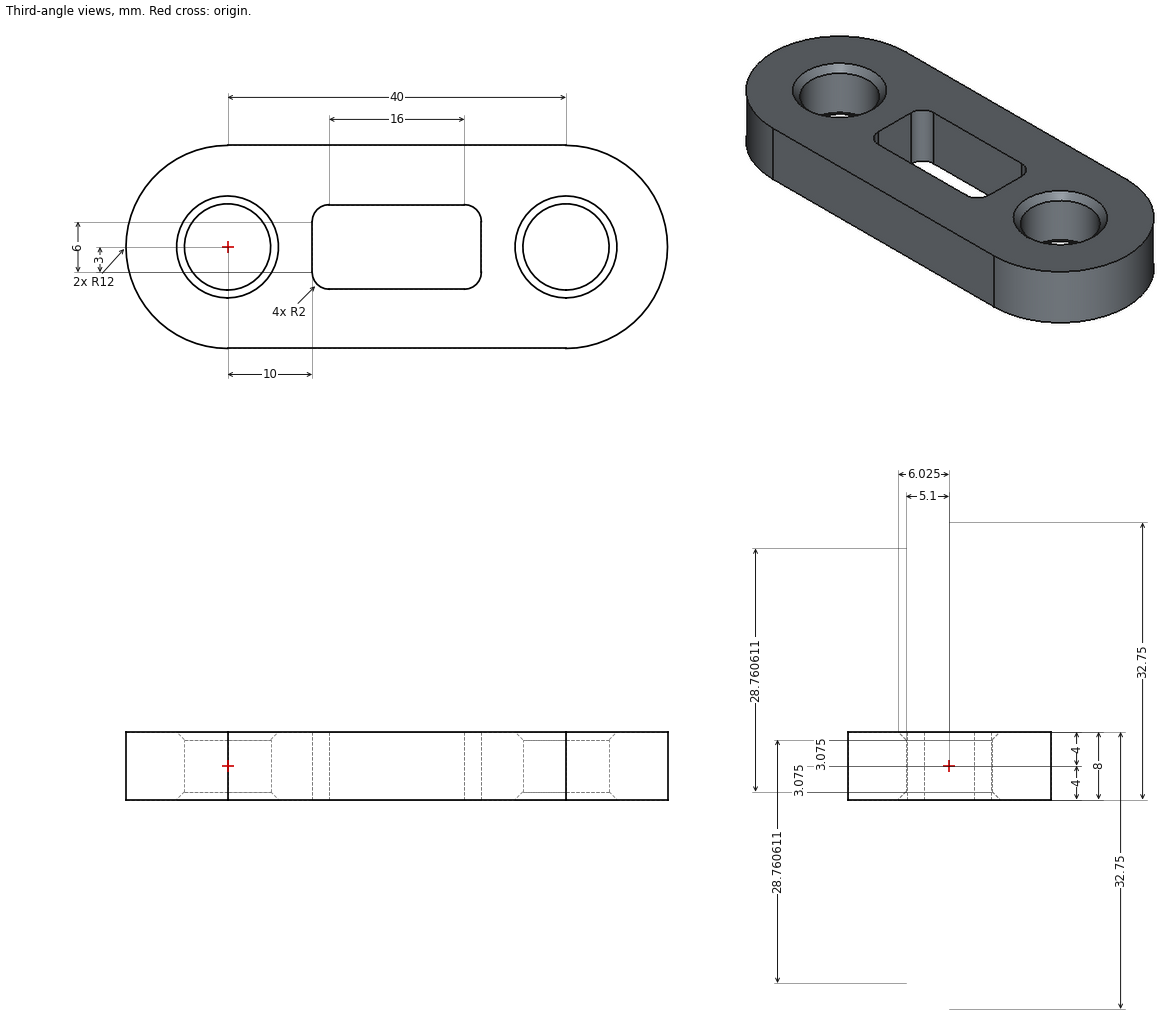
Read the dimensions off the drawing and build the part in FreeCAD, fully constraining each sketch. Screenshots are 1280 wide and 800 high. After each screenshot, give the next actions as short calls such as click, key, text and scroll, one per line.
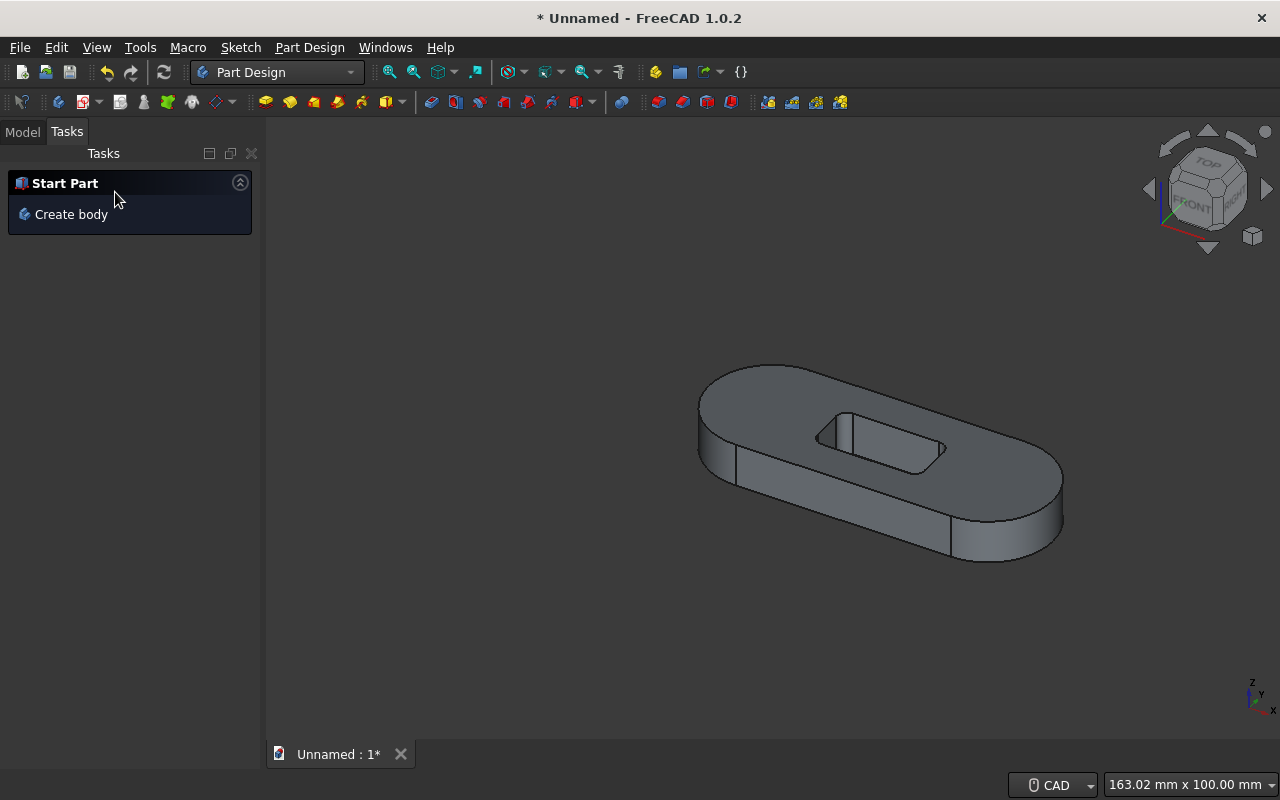
key(v)
key(f)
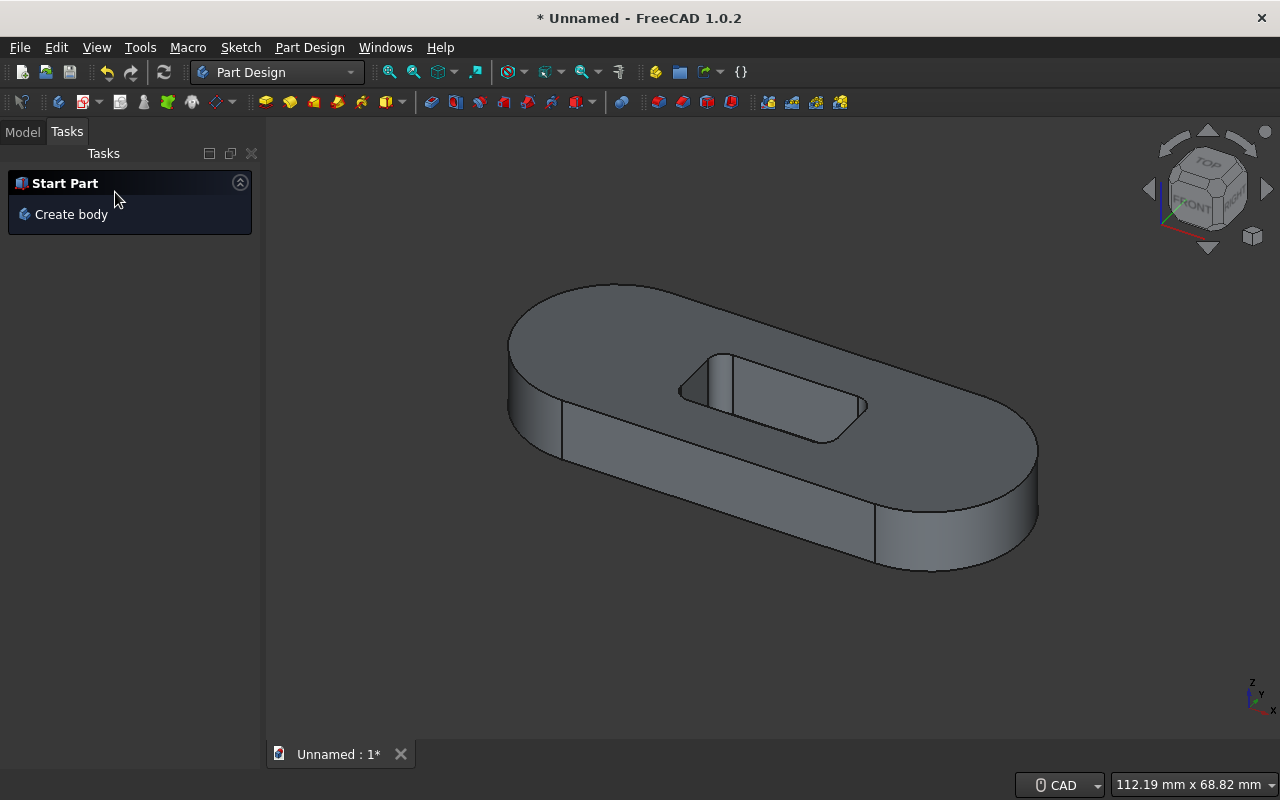
click(84, 102)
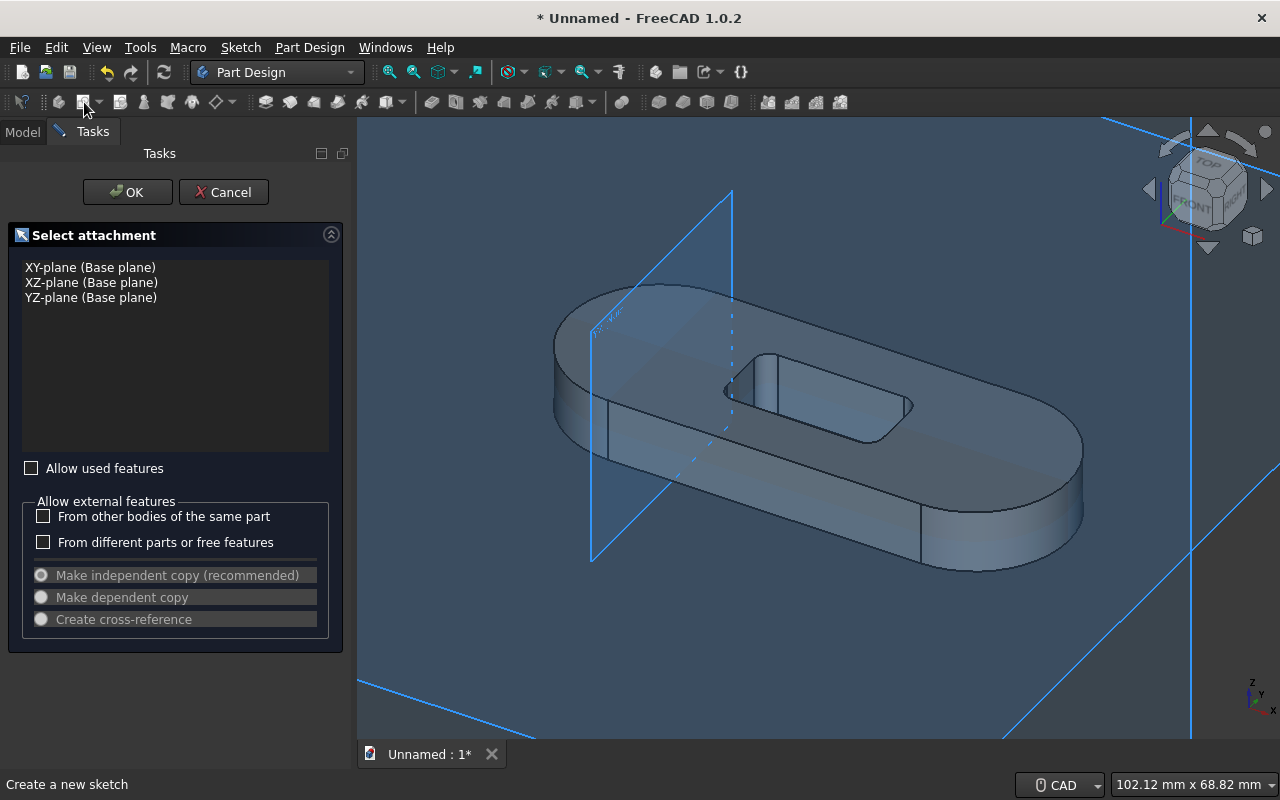
click(82, 298)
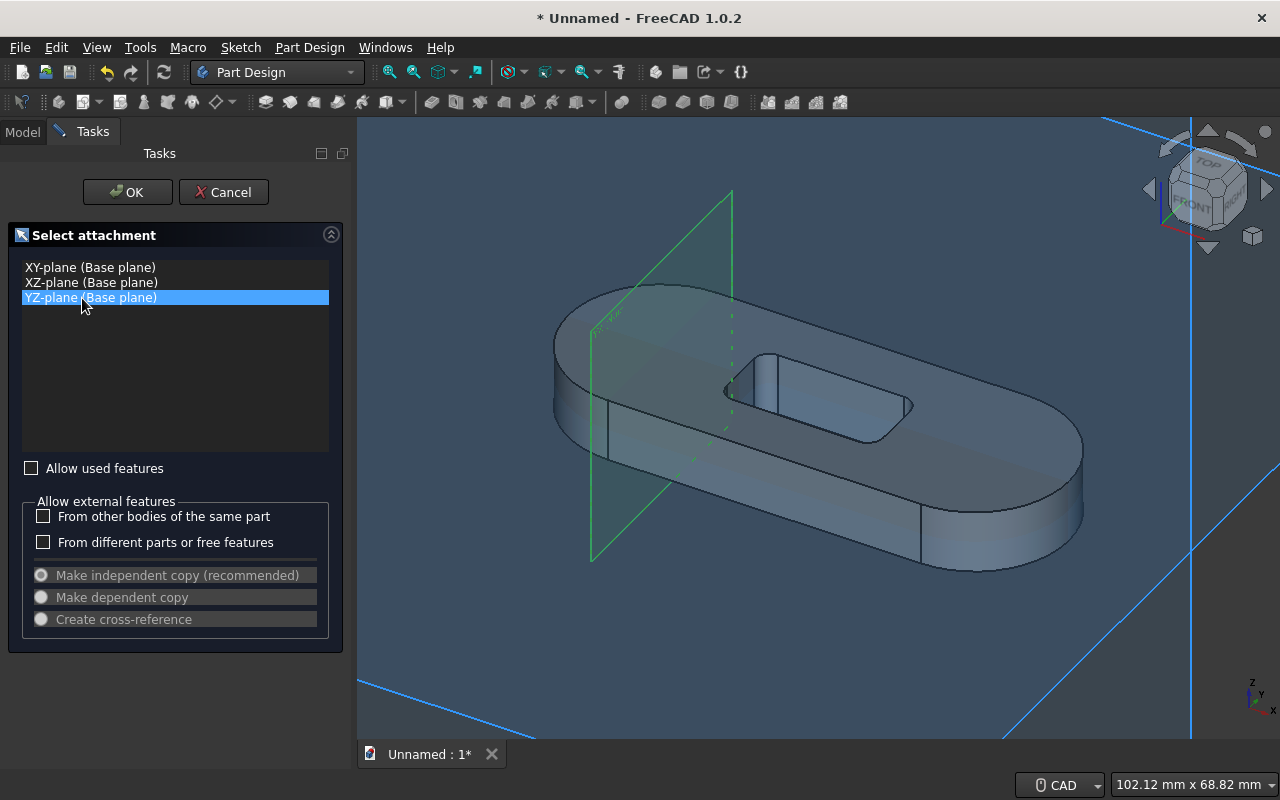
click(128, 192)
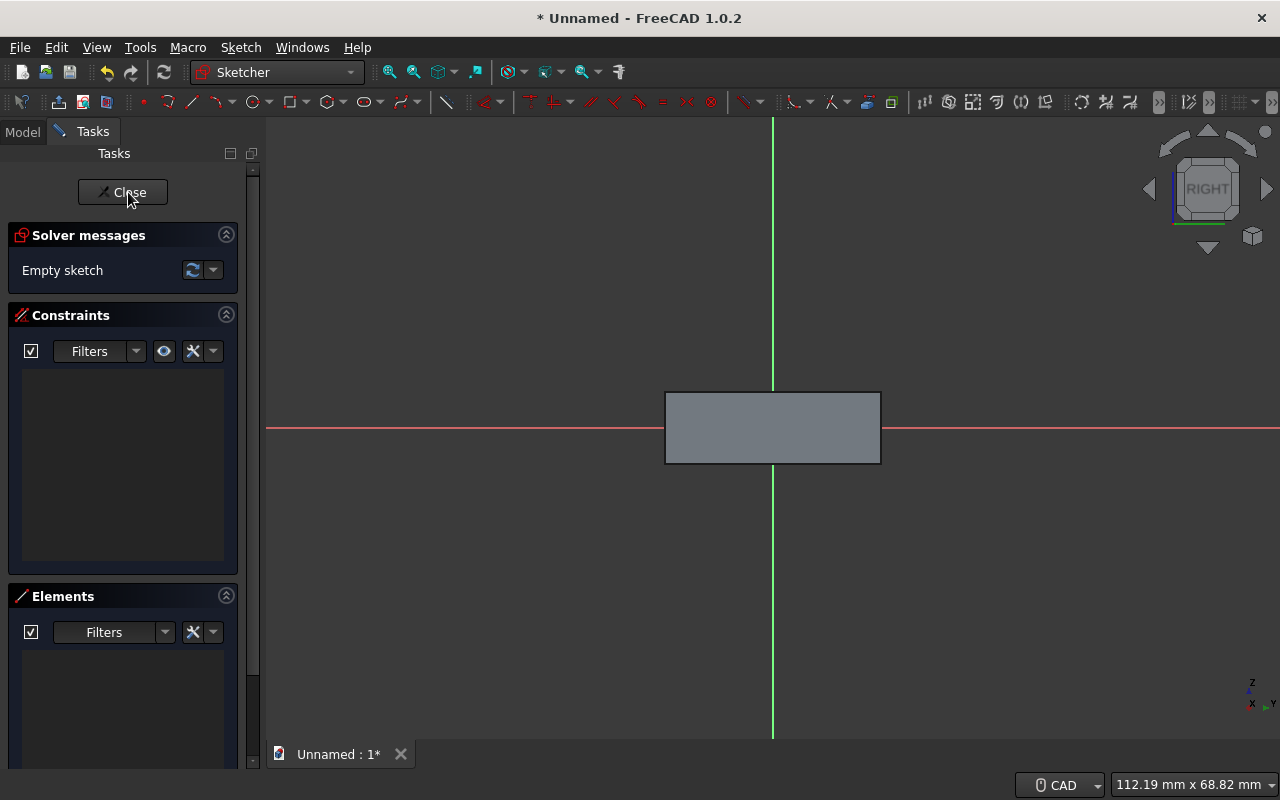
key(q)
key(s)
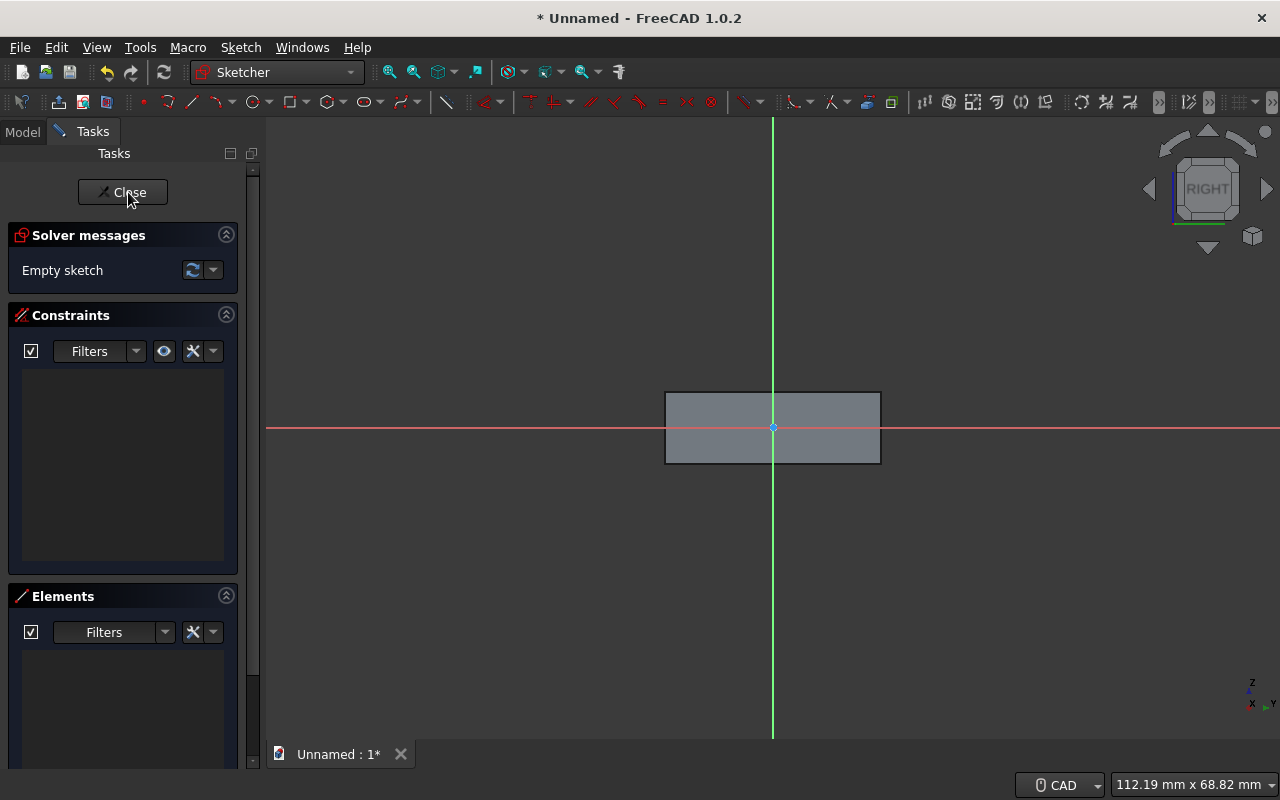
scroll(932, 711, up, 1)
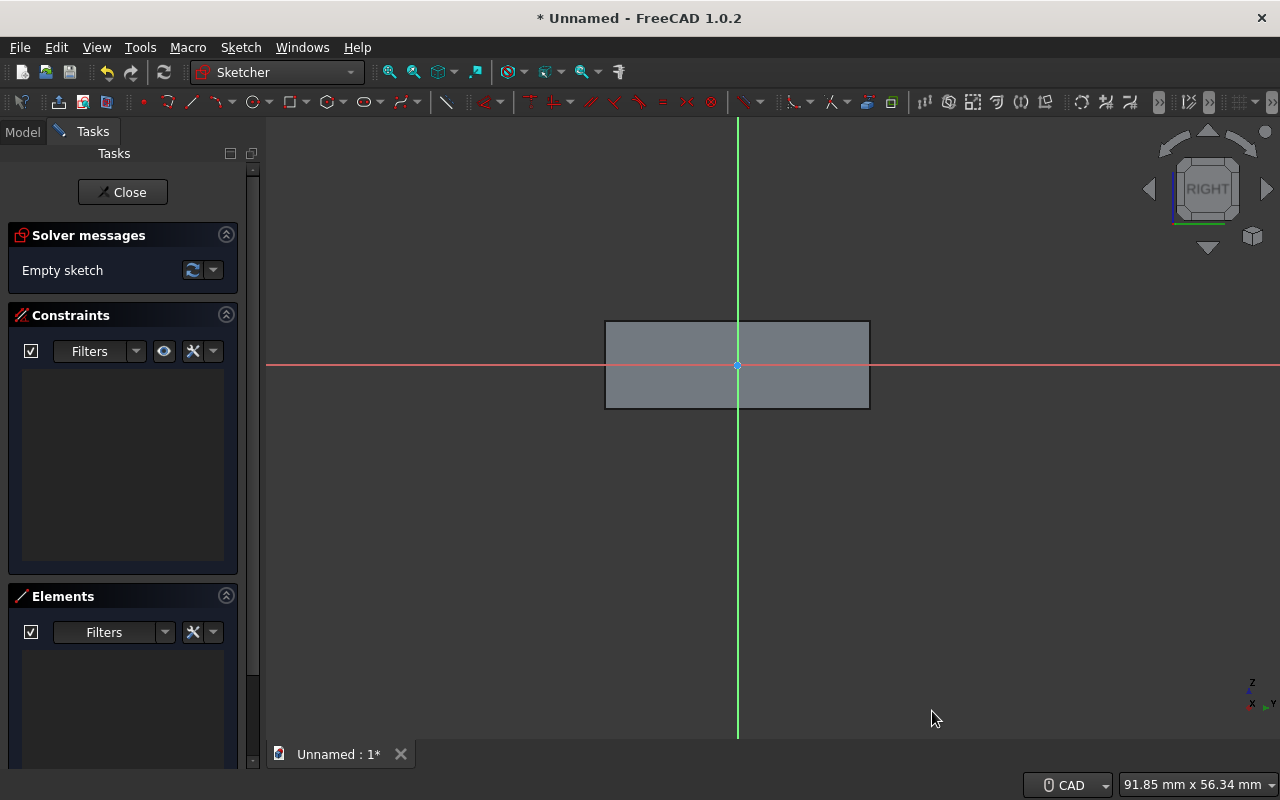
click(168, 102)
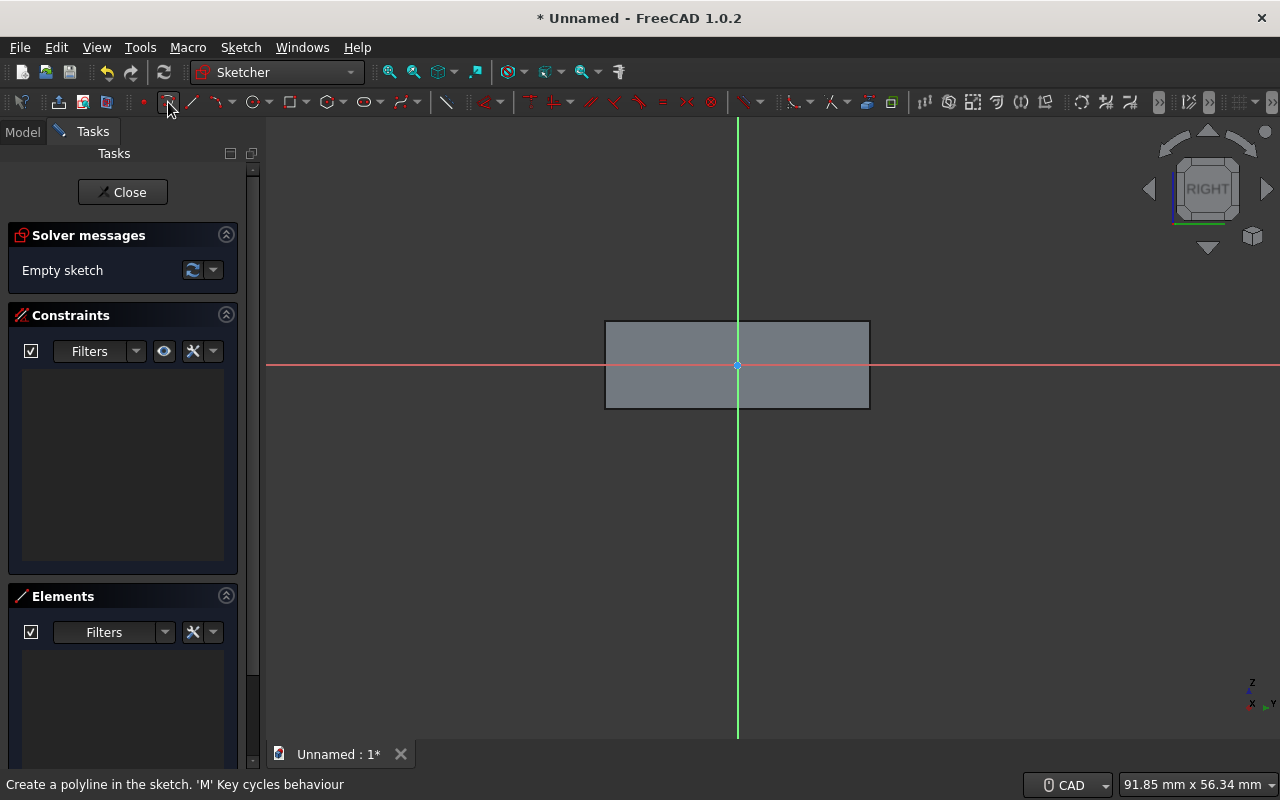
click(738, 321)
click(671, 321)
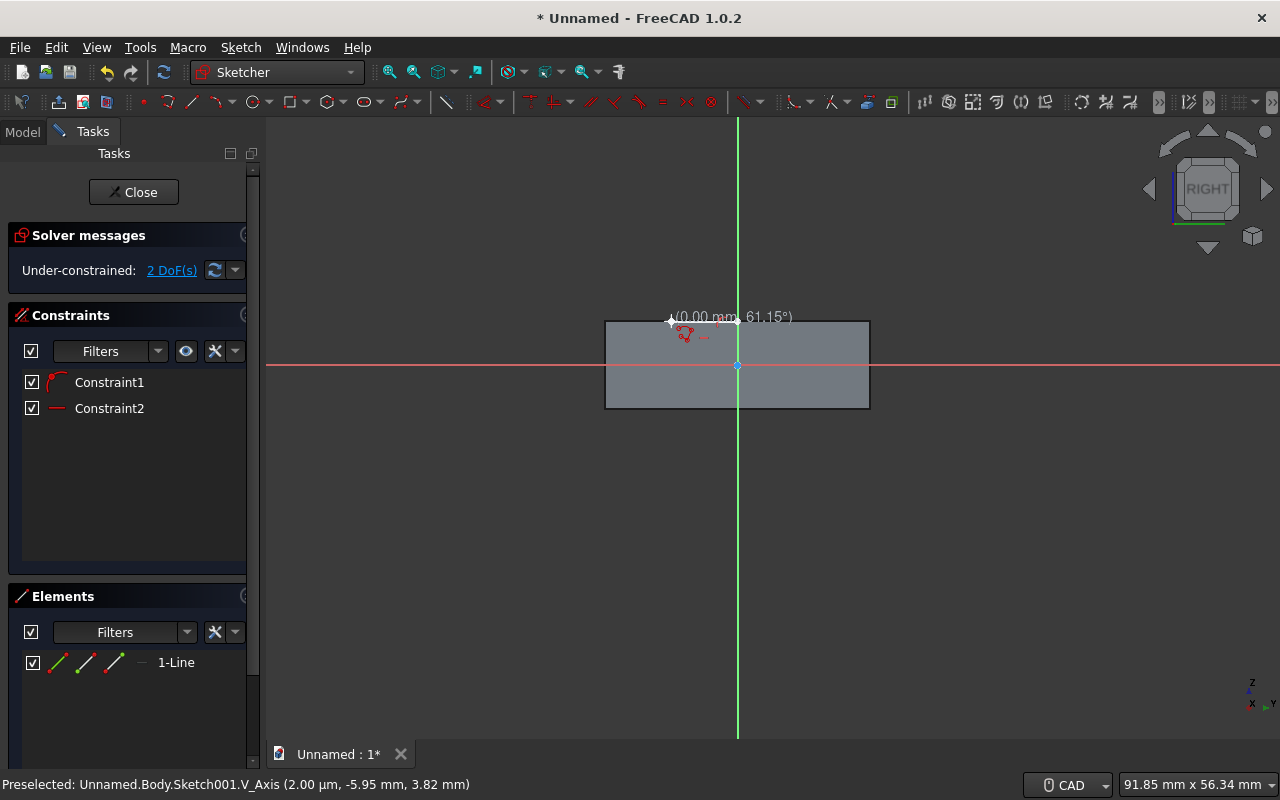
scroll(681, 331, up, 3)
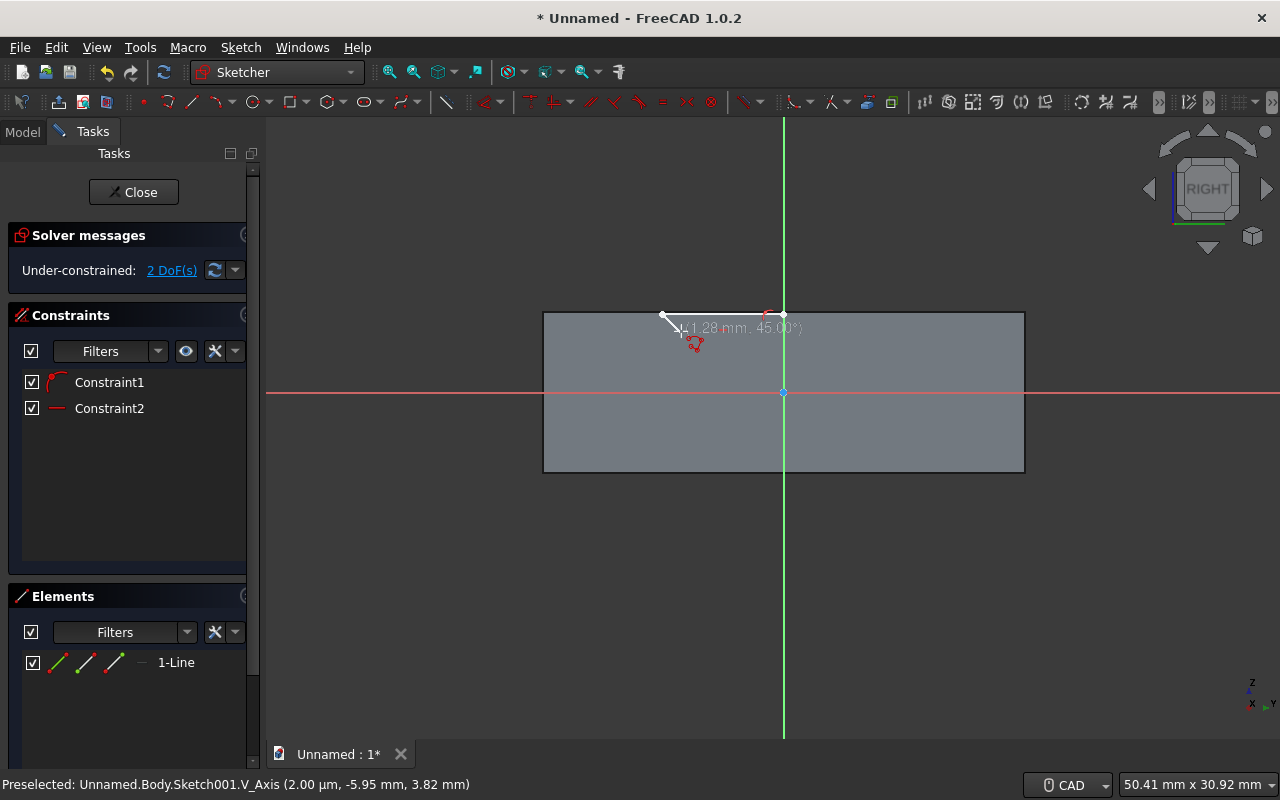
click(681, 331)